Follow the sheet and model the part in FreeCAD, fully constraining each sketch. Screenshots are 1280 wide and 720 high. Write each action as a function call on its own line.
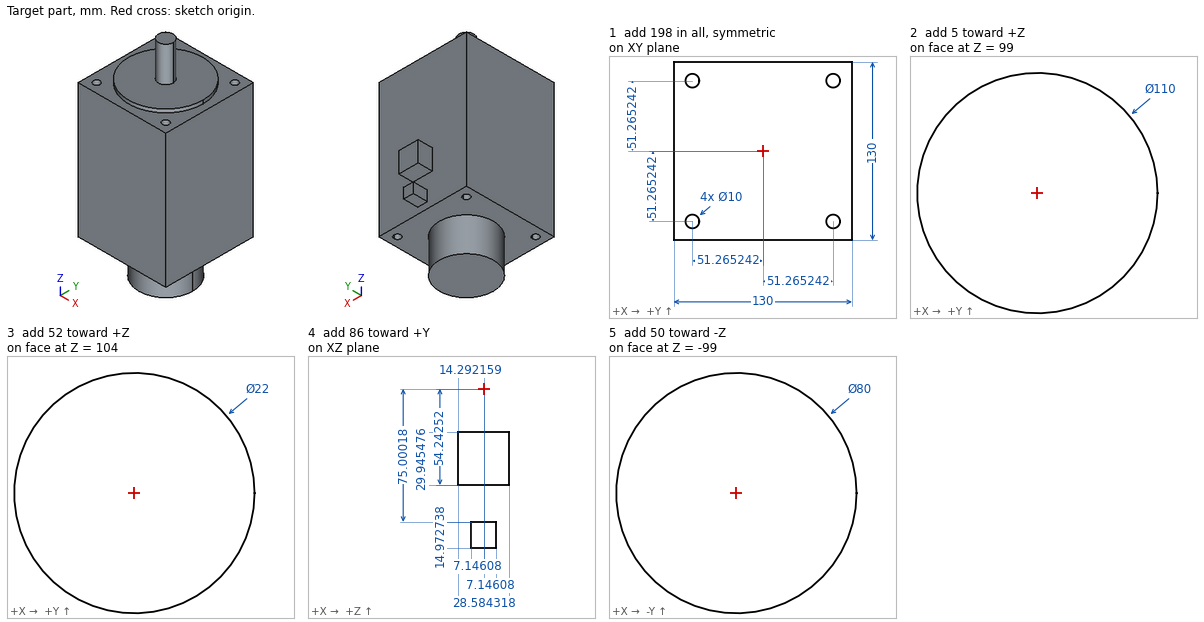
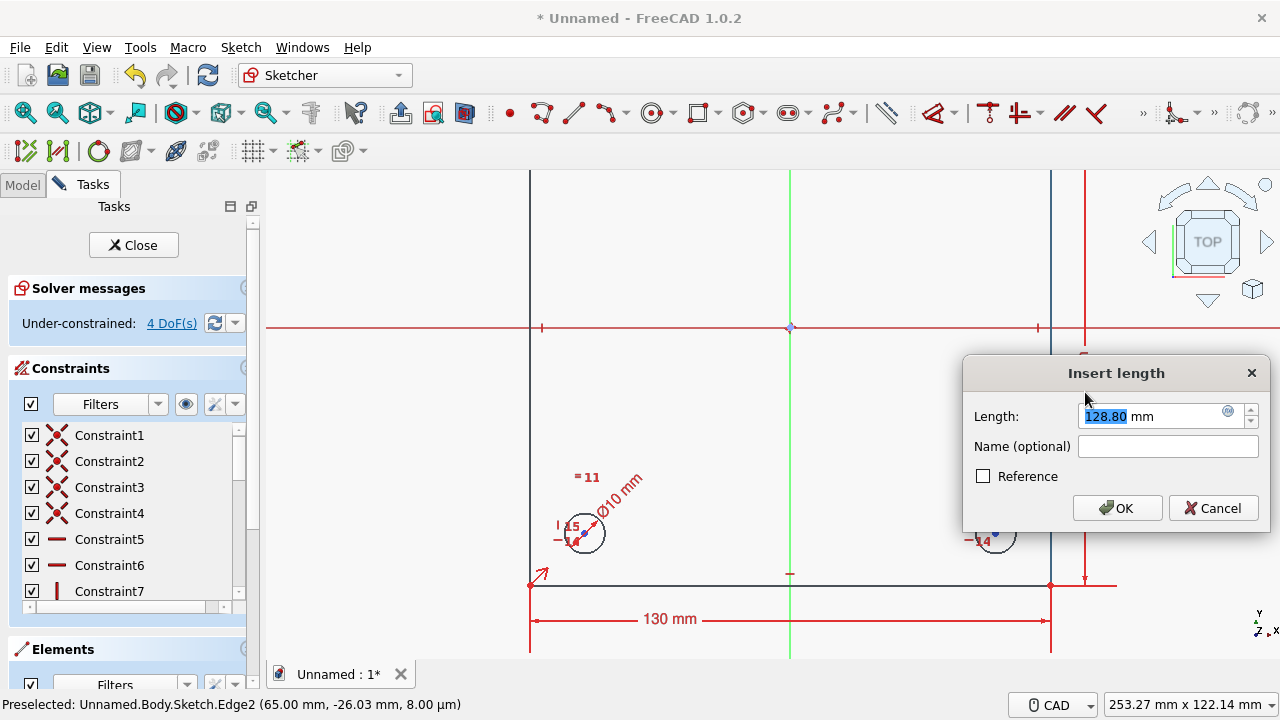
text(130)
key(Return)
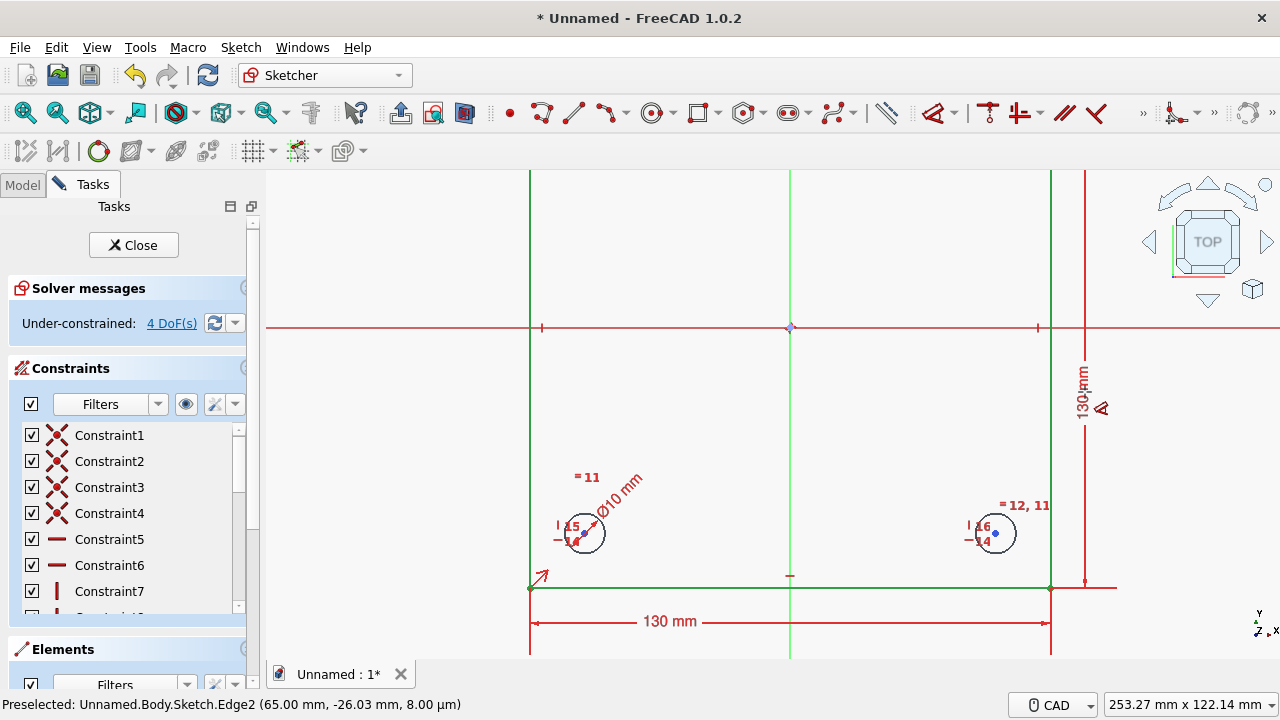
click(585, 534)
click(688, 568)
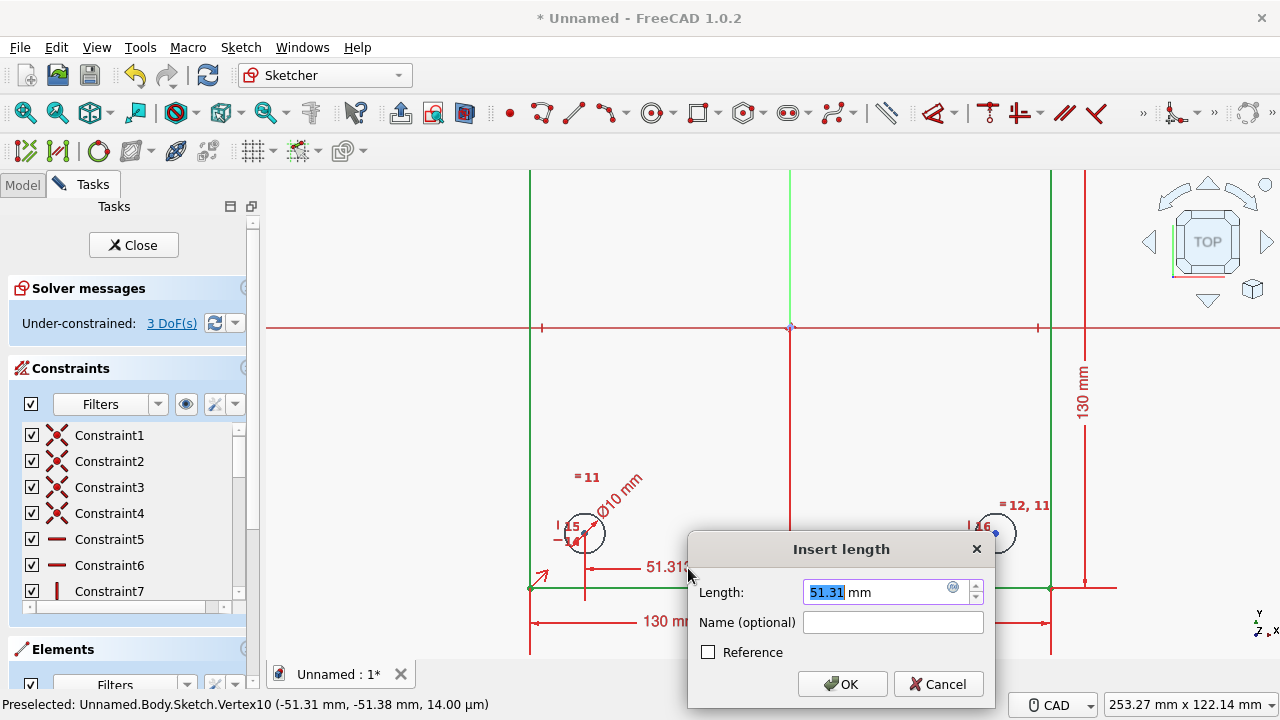
text(51.265242)
key(Return)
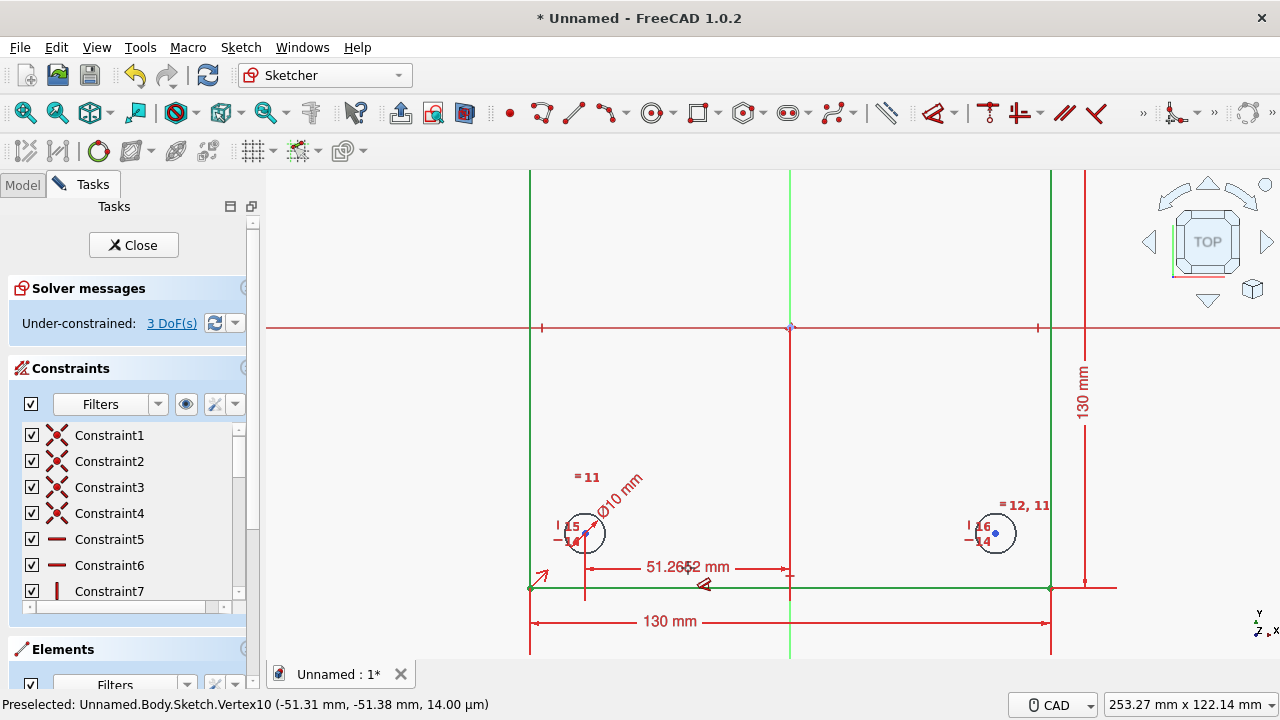
click(585, 534)
click(551, 431)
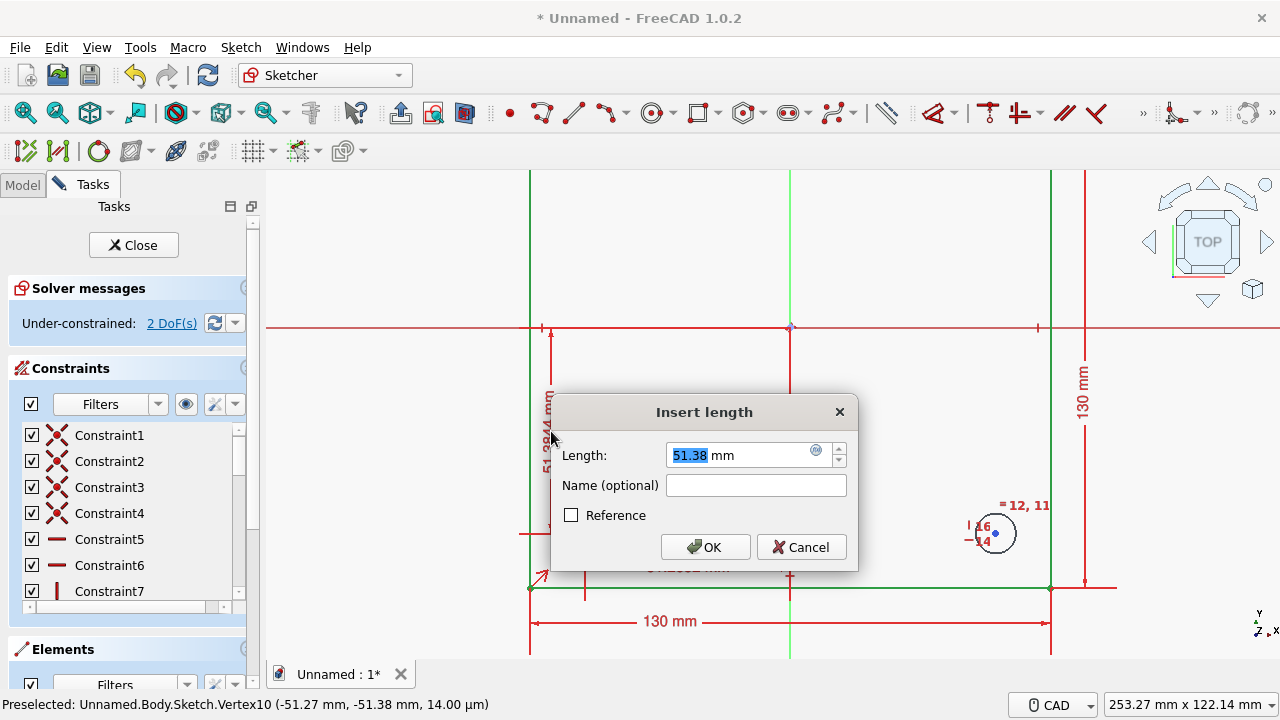
text(51.265242)
key(Return)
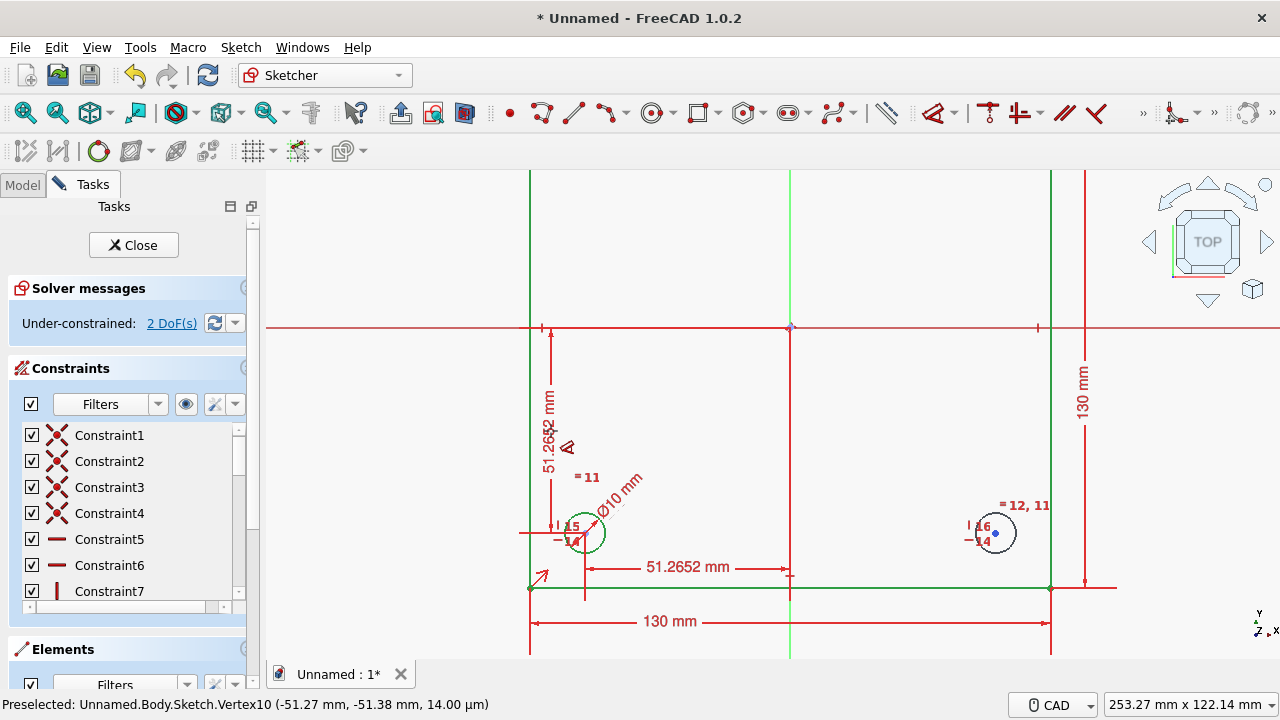
click(996, 533)
click(893, 567)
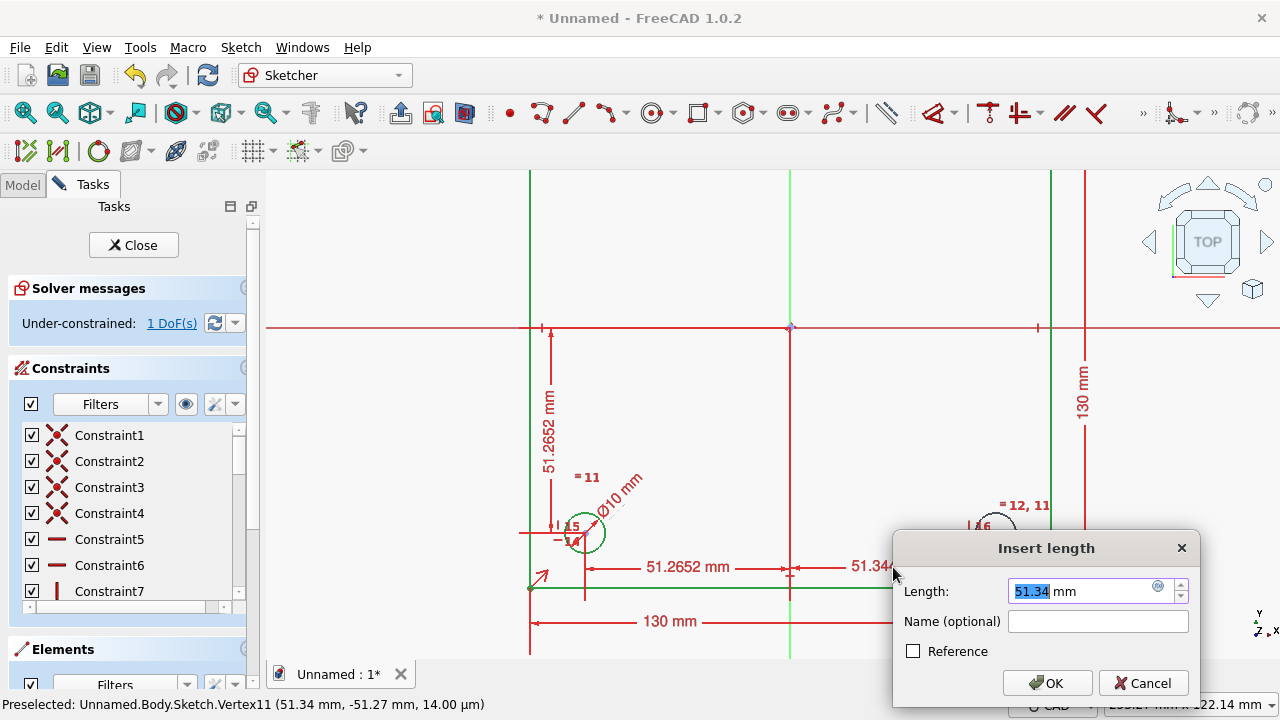
text(51.265242)
key(Return)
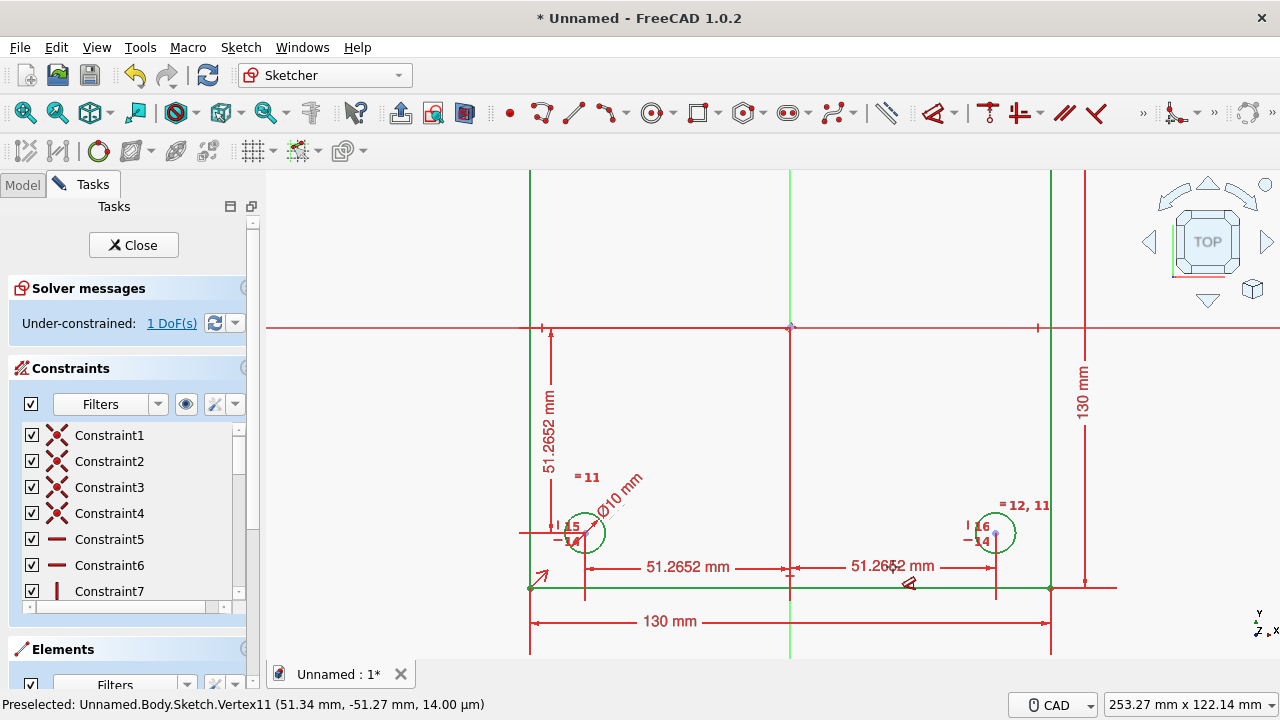
scroll(600, 520, down, 3)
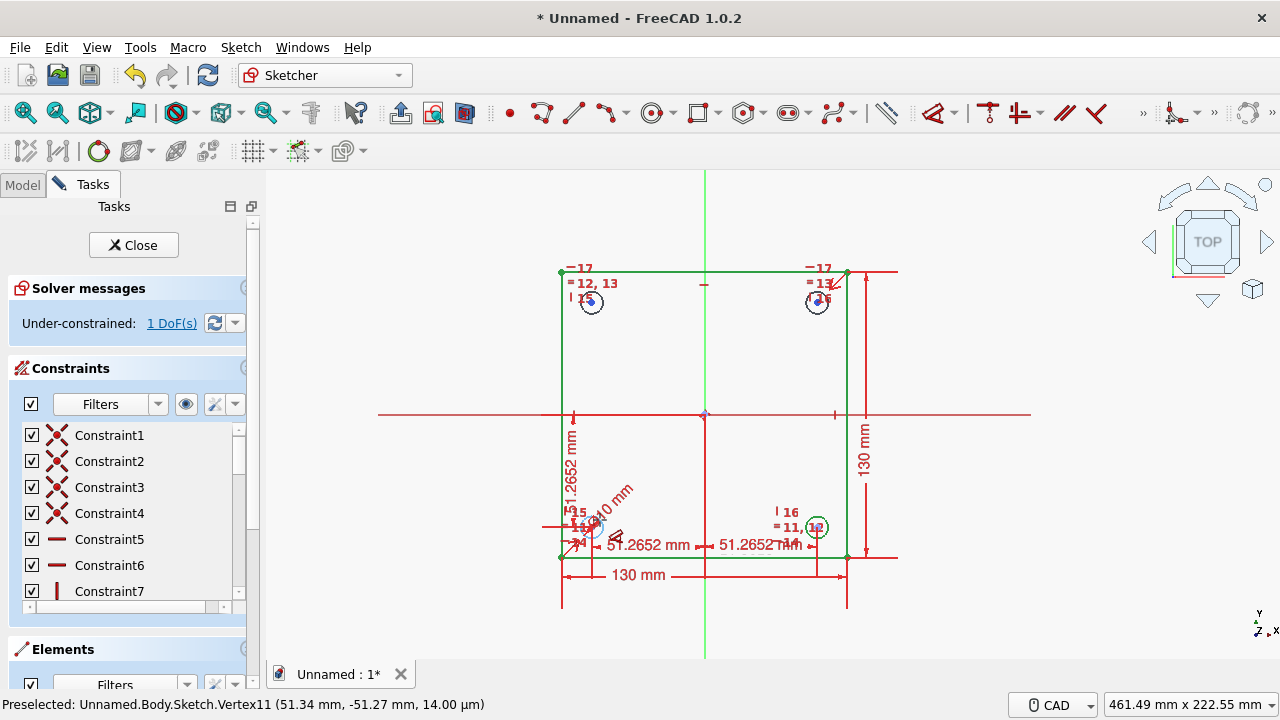
click(592, 303)
click(739, 359)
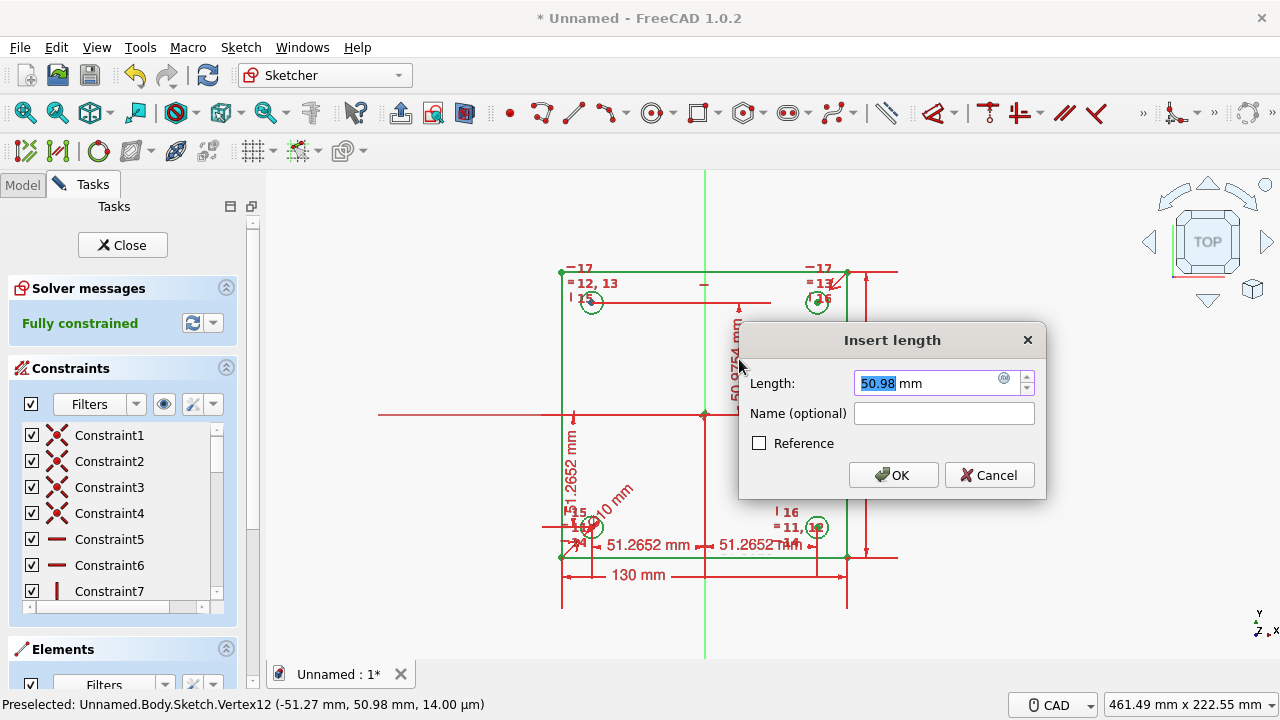
text(51.265242)
key(Return)
key(Escape)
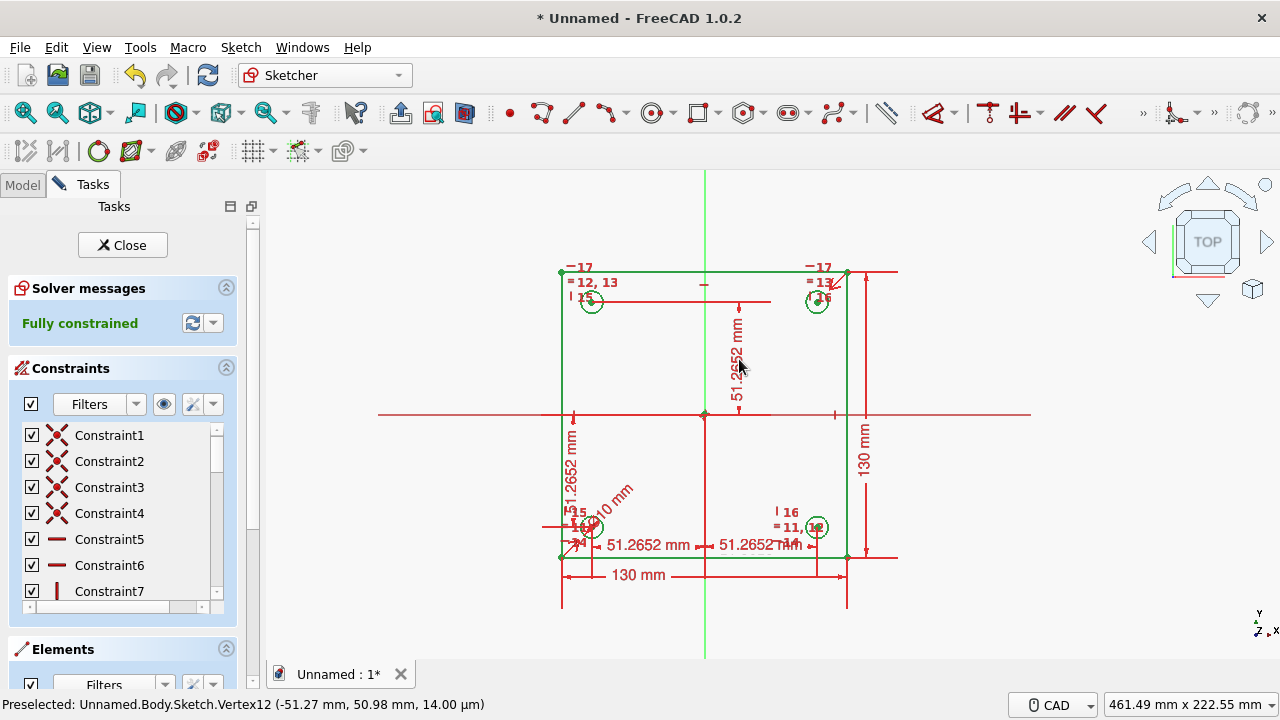
click(123, 245)